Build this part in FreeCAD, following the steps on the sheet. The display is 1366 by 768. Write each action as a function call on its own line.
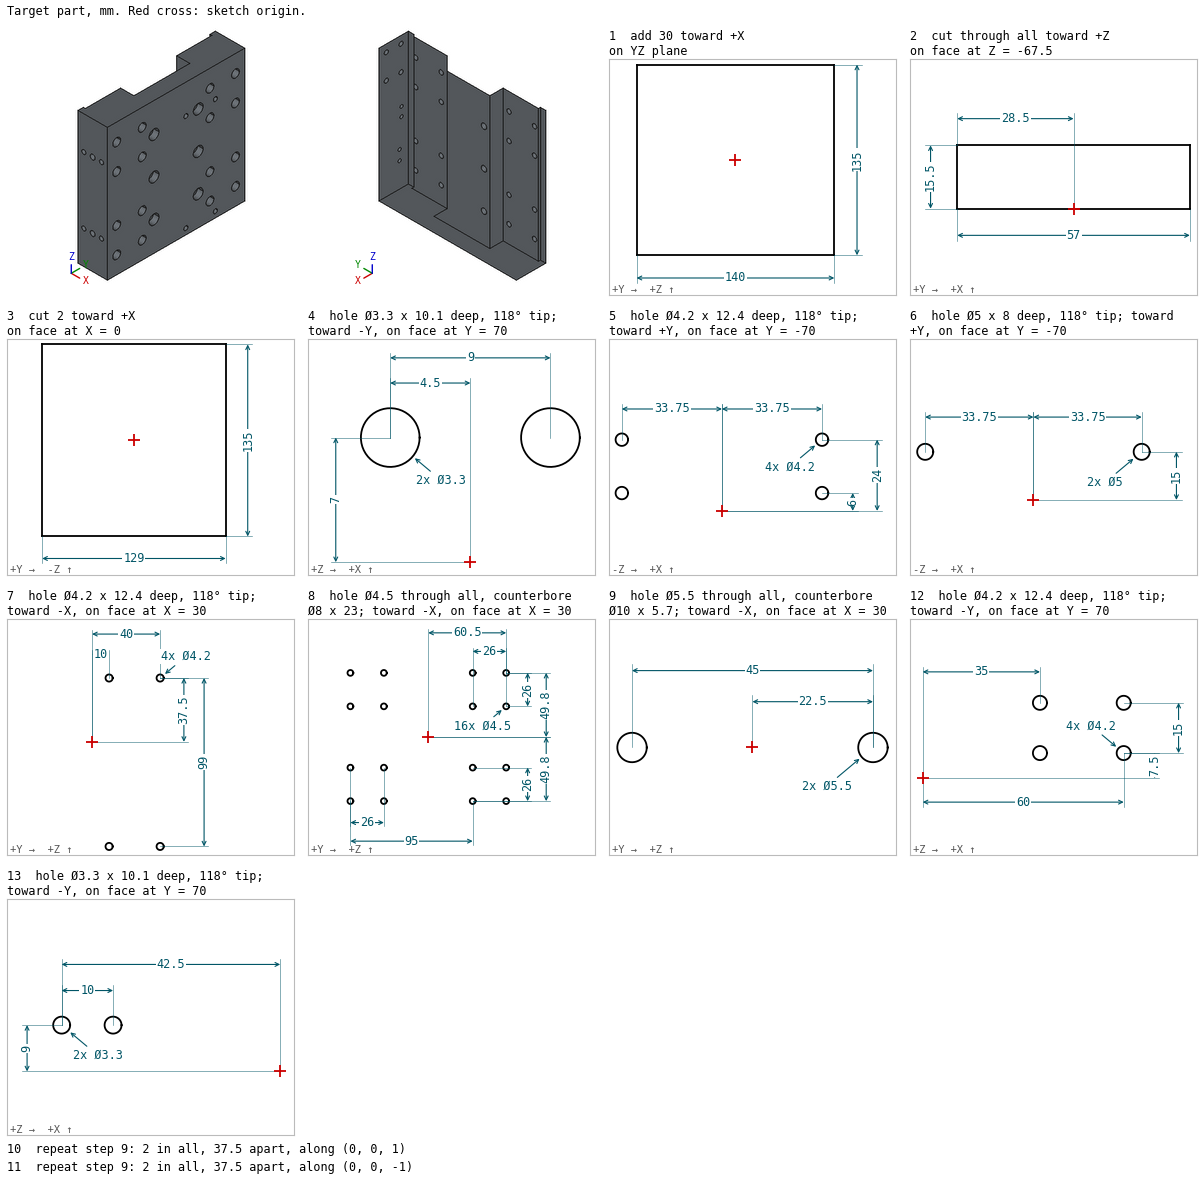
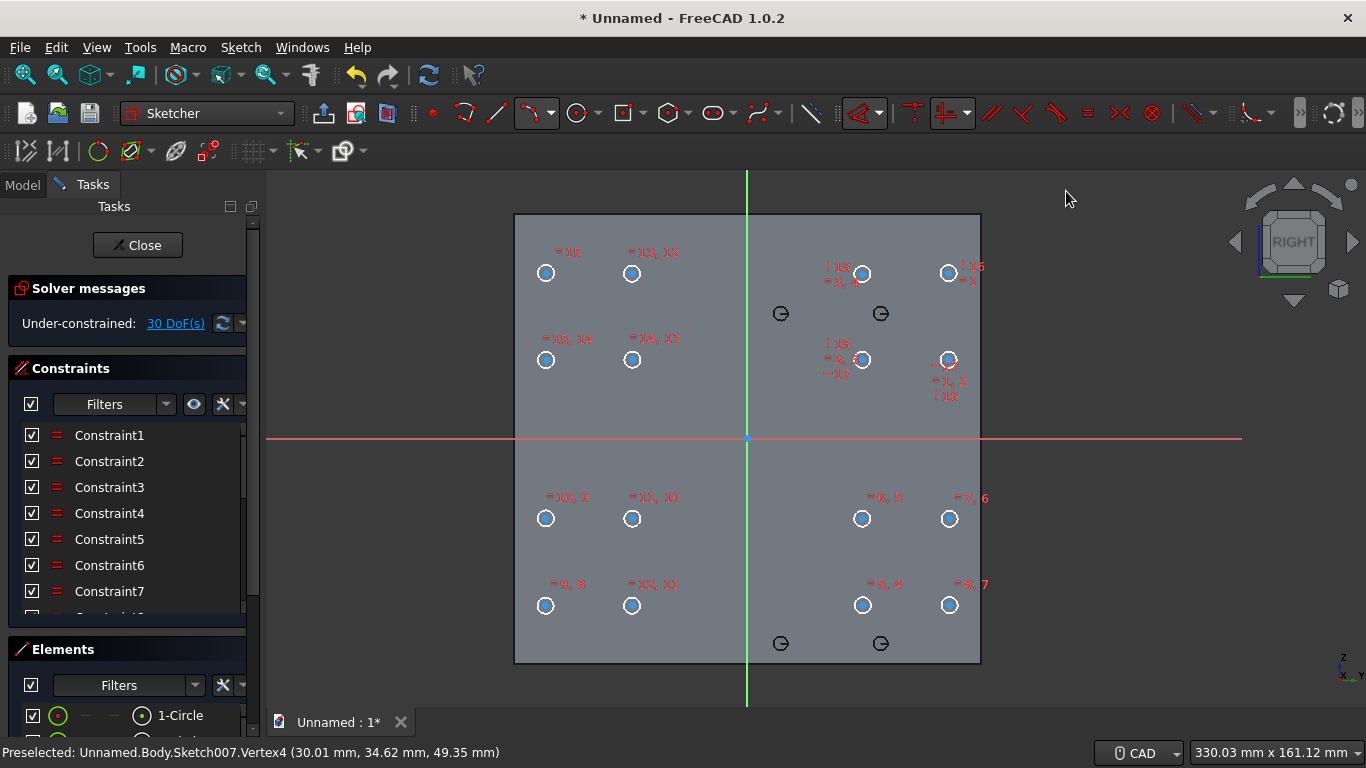
click(949, 273)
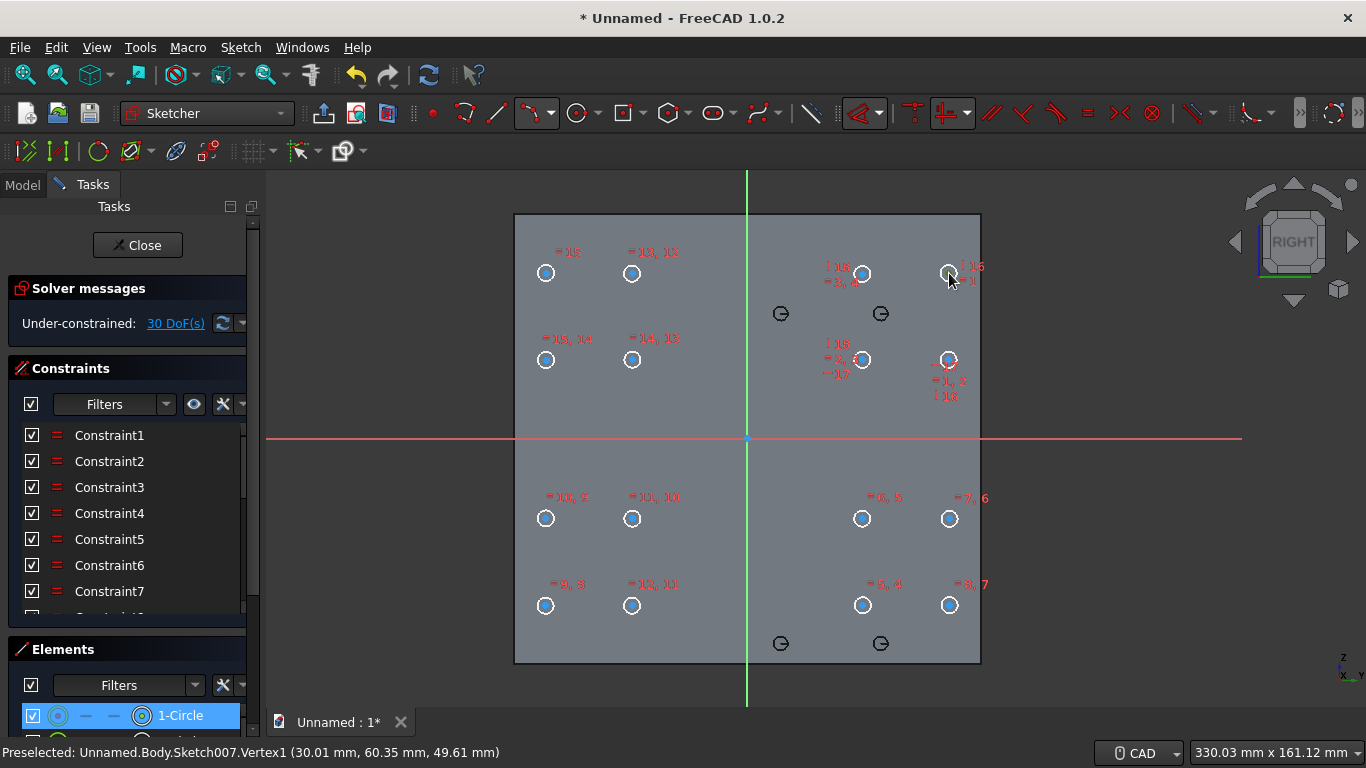
click(862, 274)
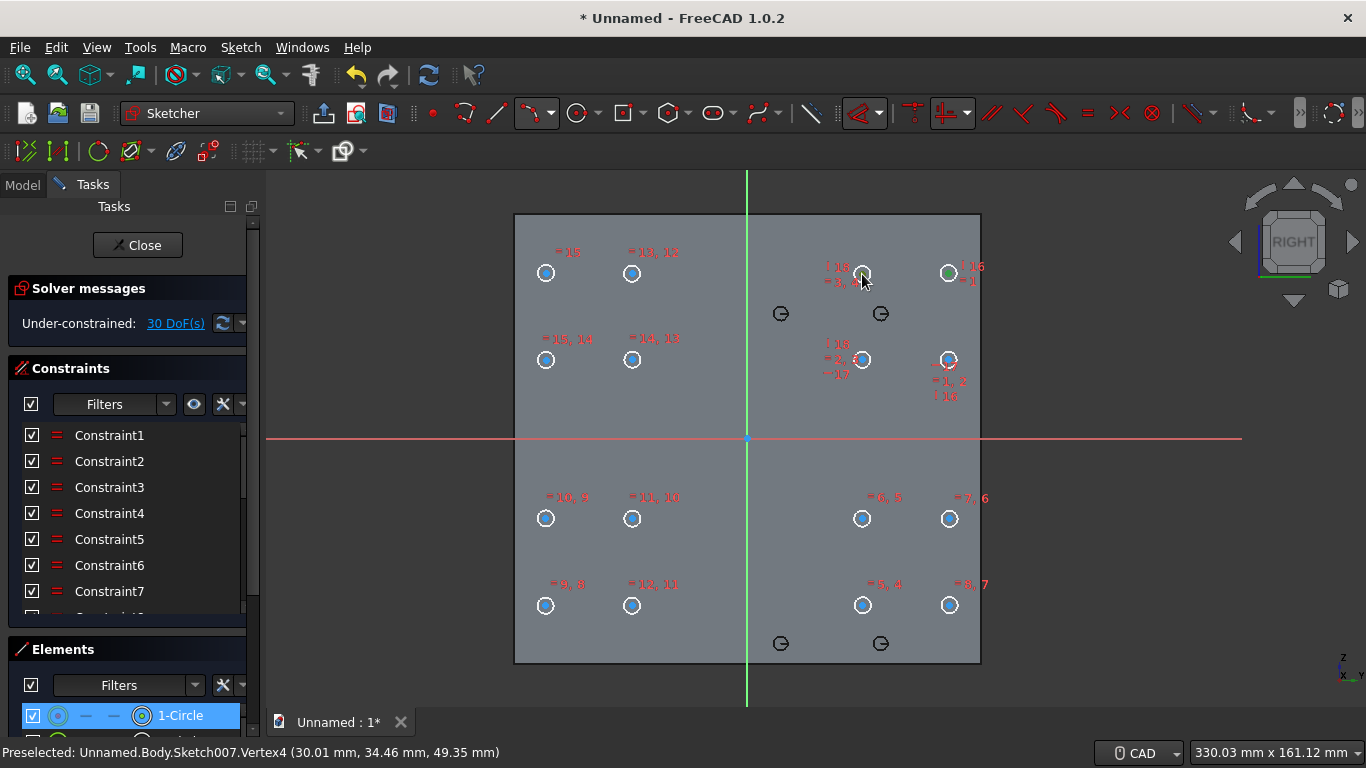
click(970, 114)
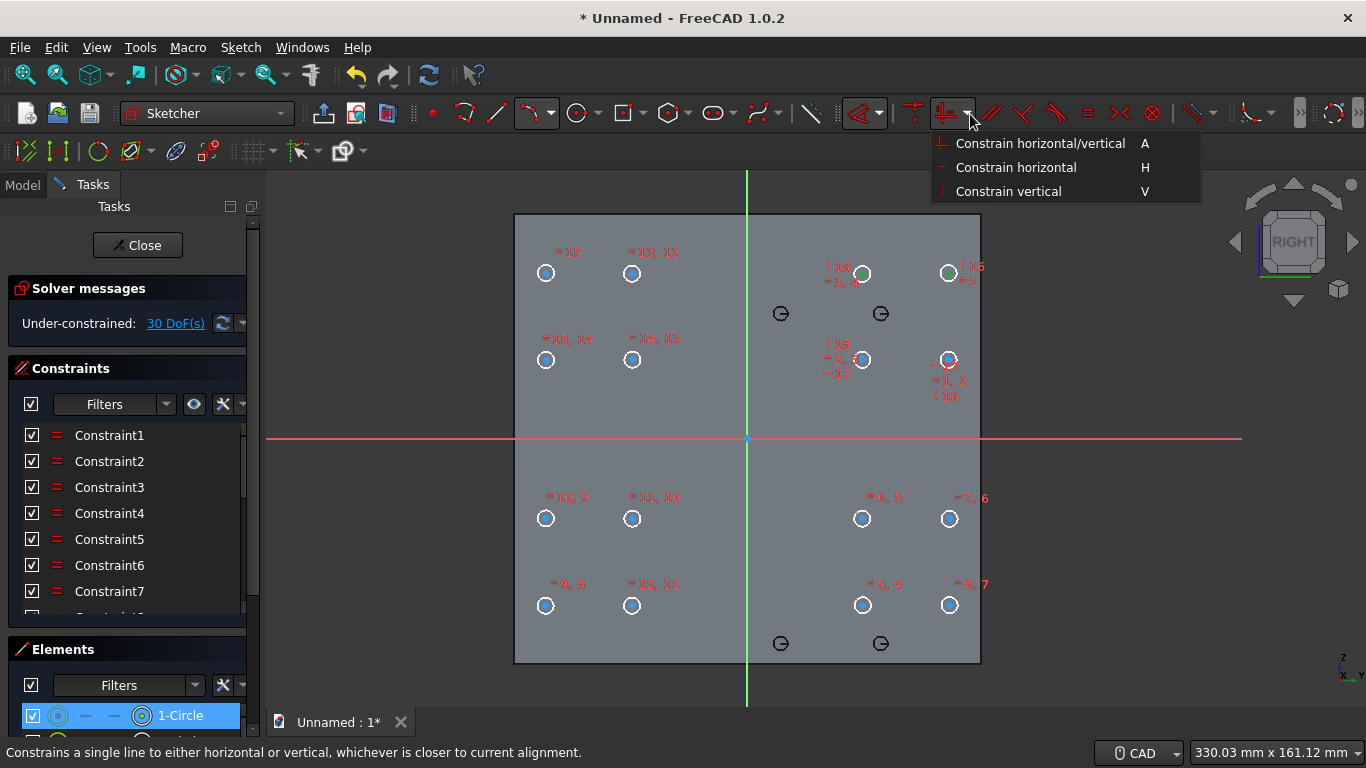
click(1066, 167)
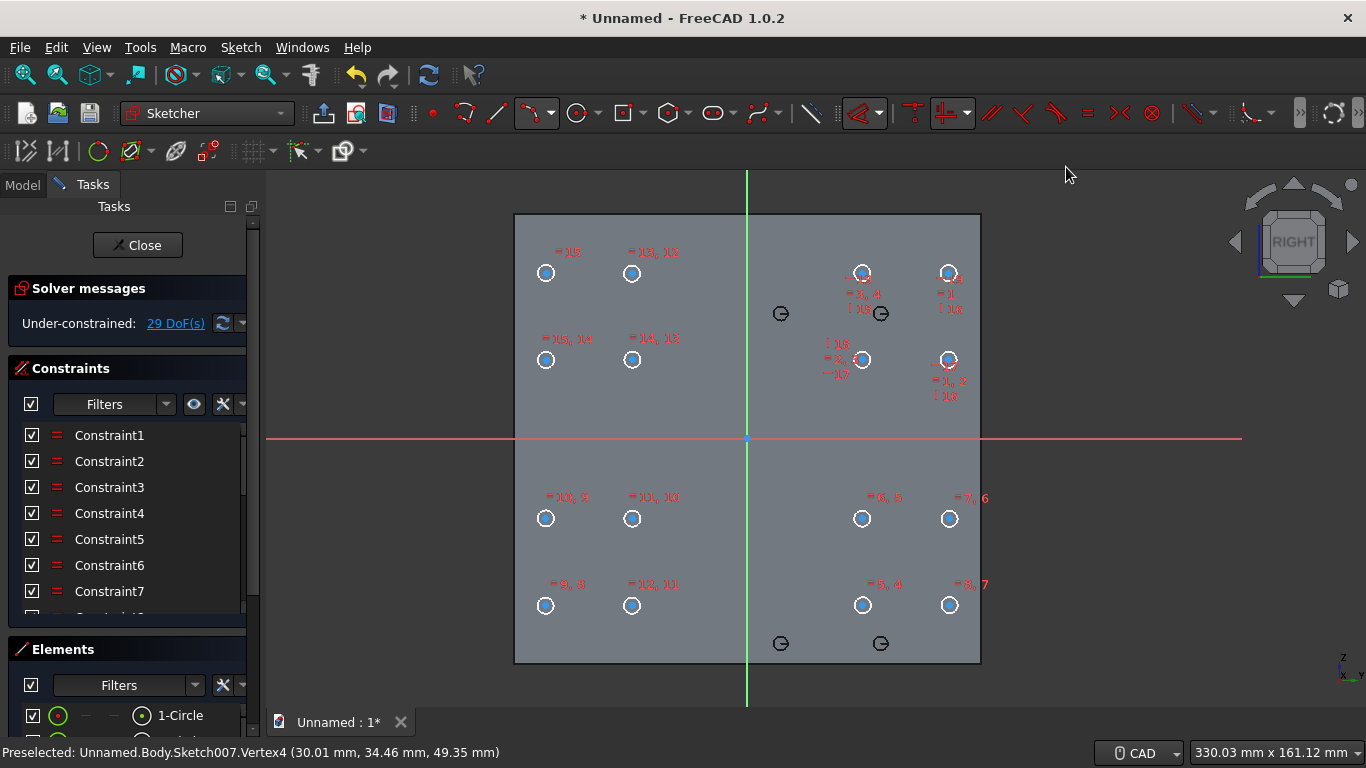
click(862, 360)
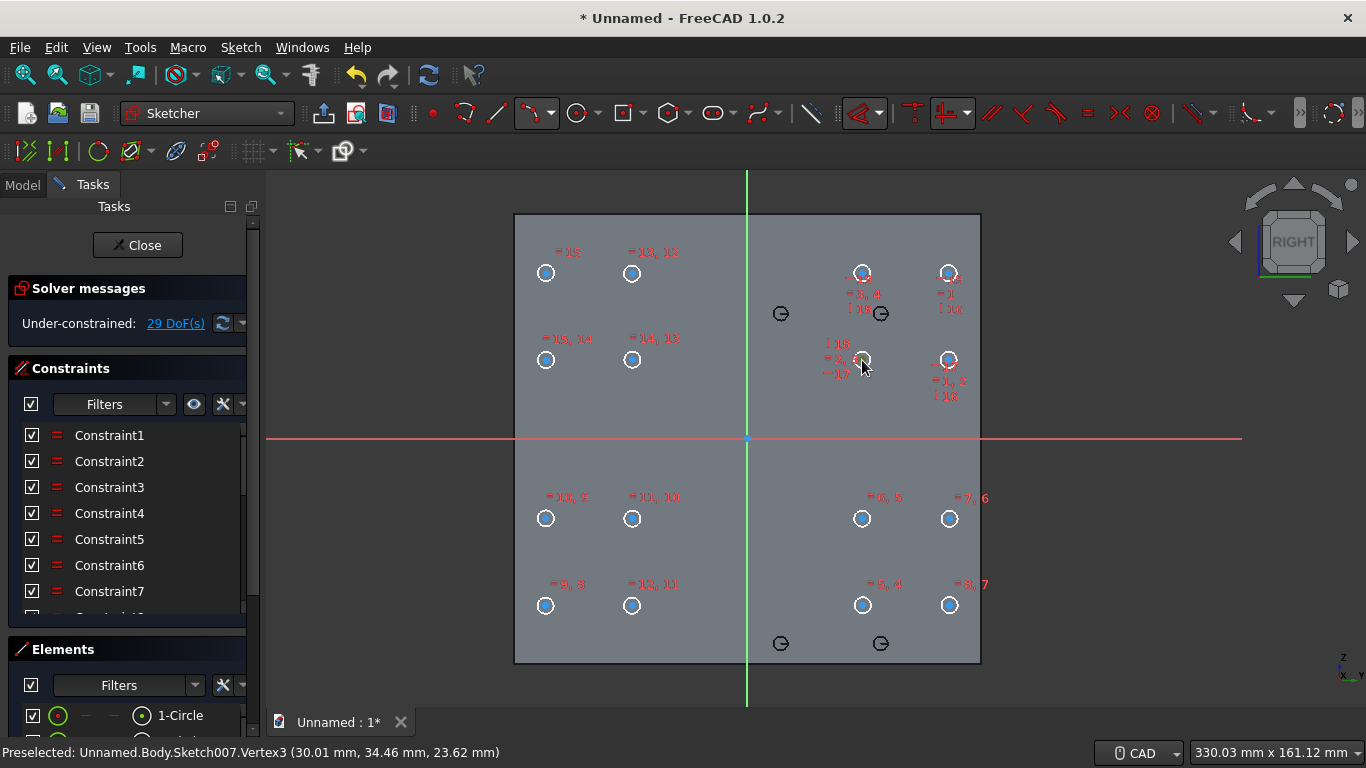
click(863, 605)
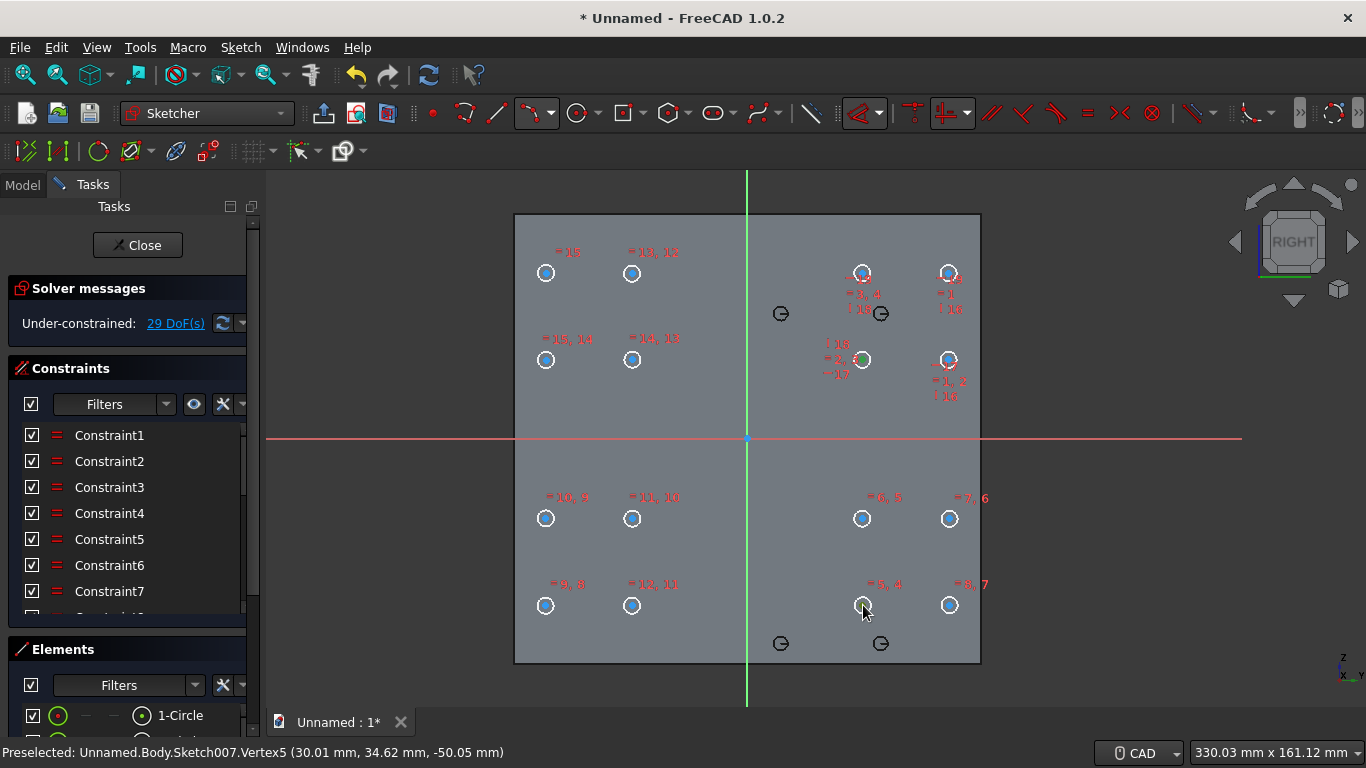
click(970, 114)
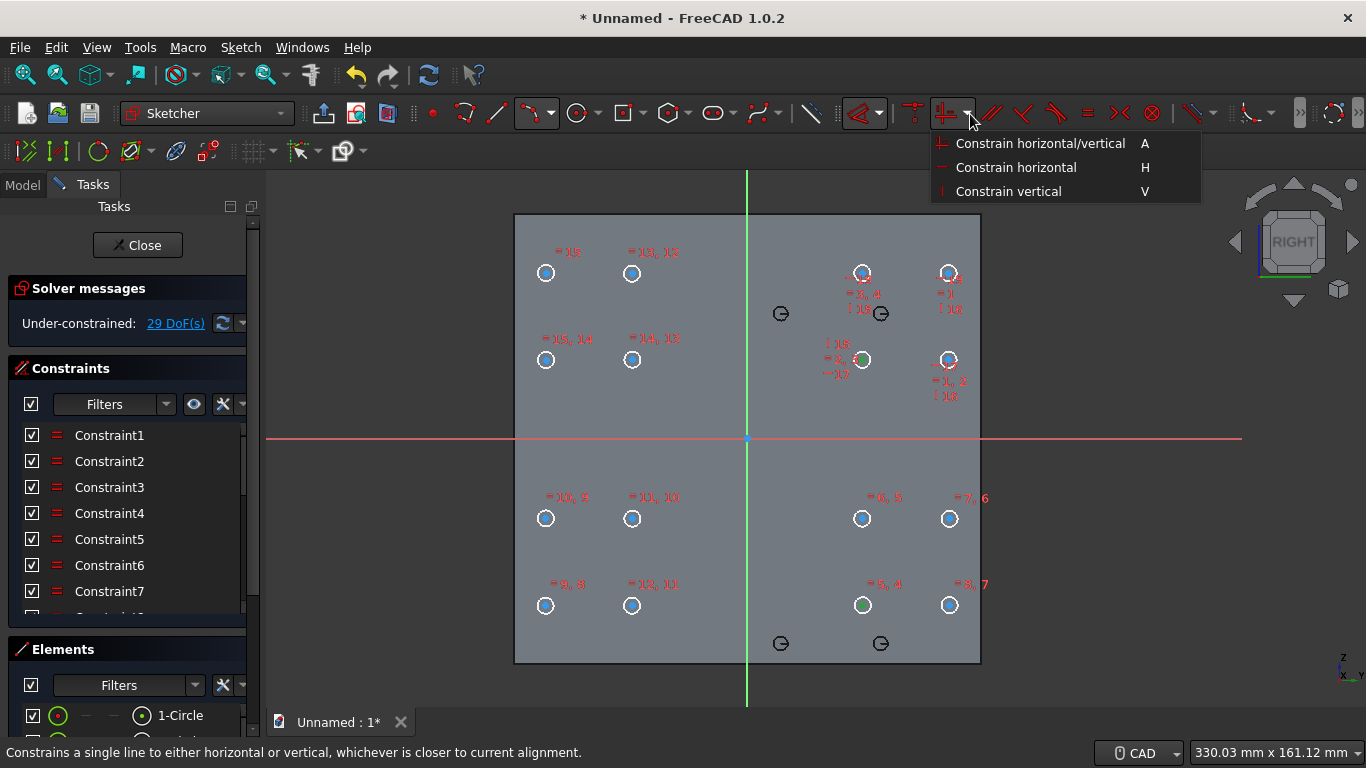
click(1066, 191)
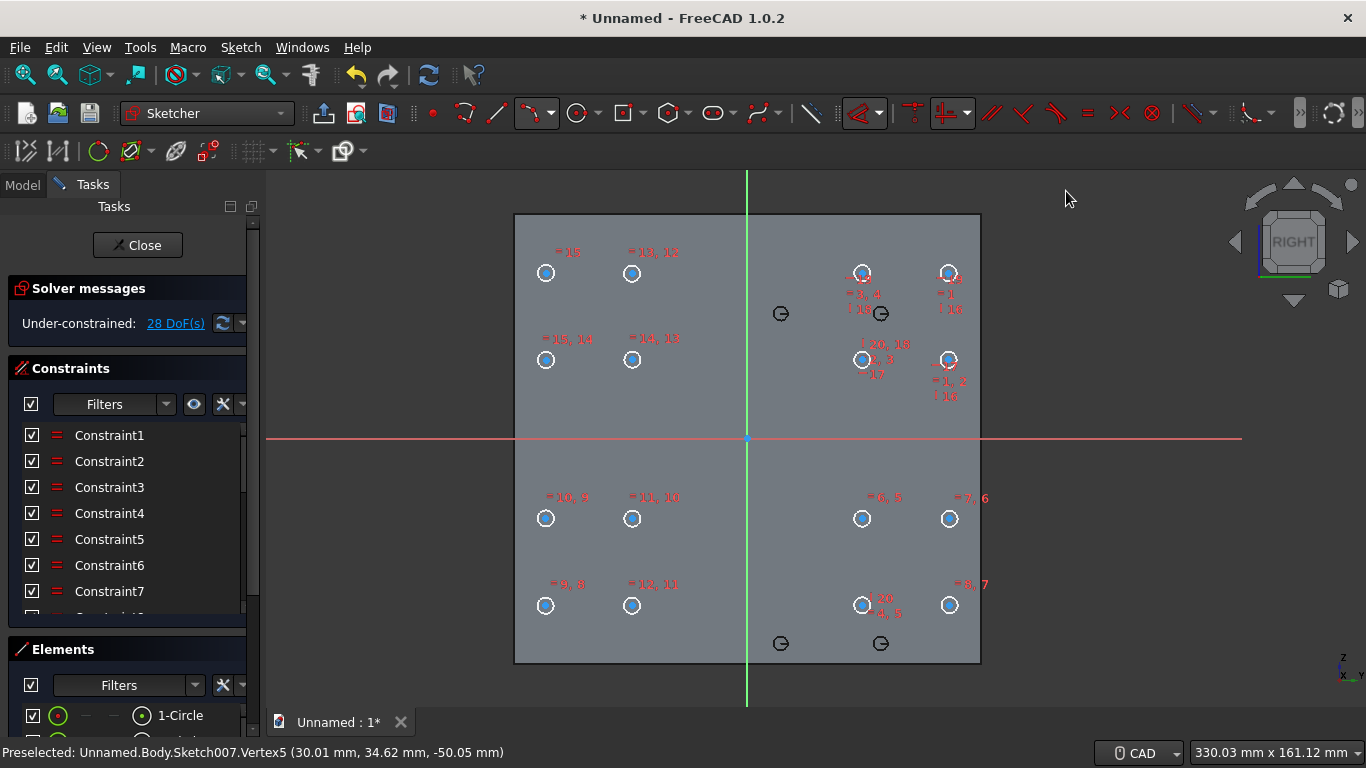
click(862, 605)